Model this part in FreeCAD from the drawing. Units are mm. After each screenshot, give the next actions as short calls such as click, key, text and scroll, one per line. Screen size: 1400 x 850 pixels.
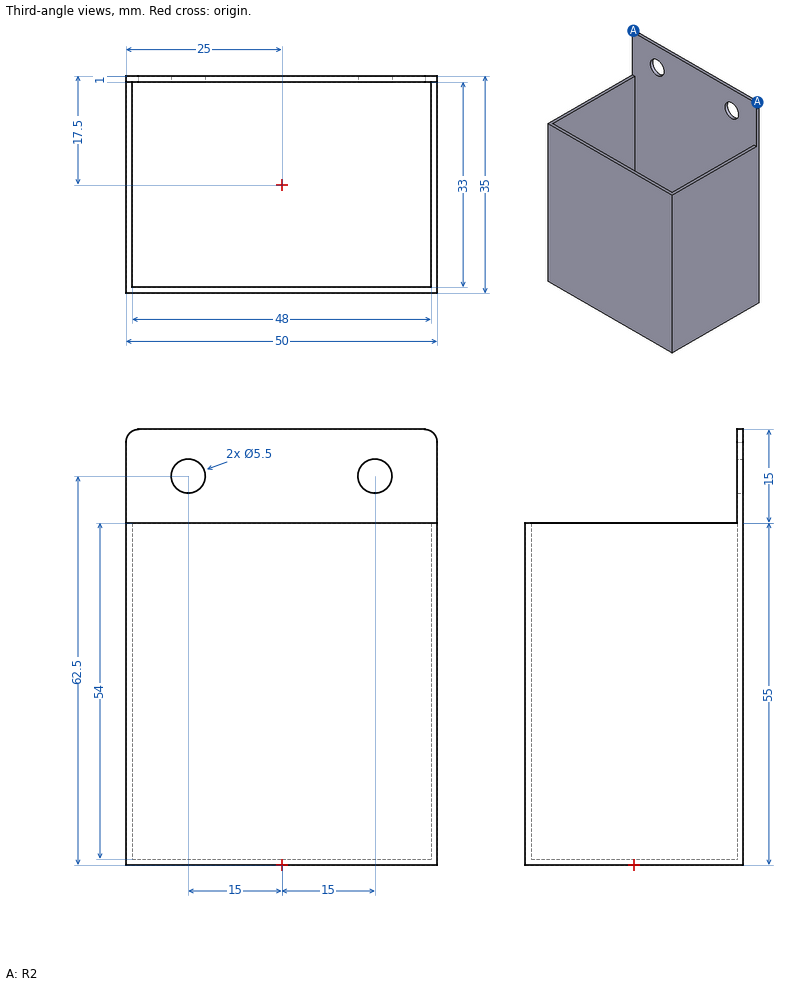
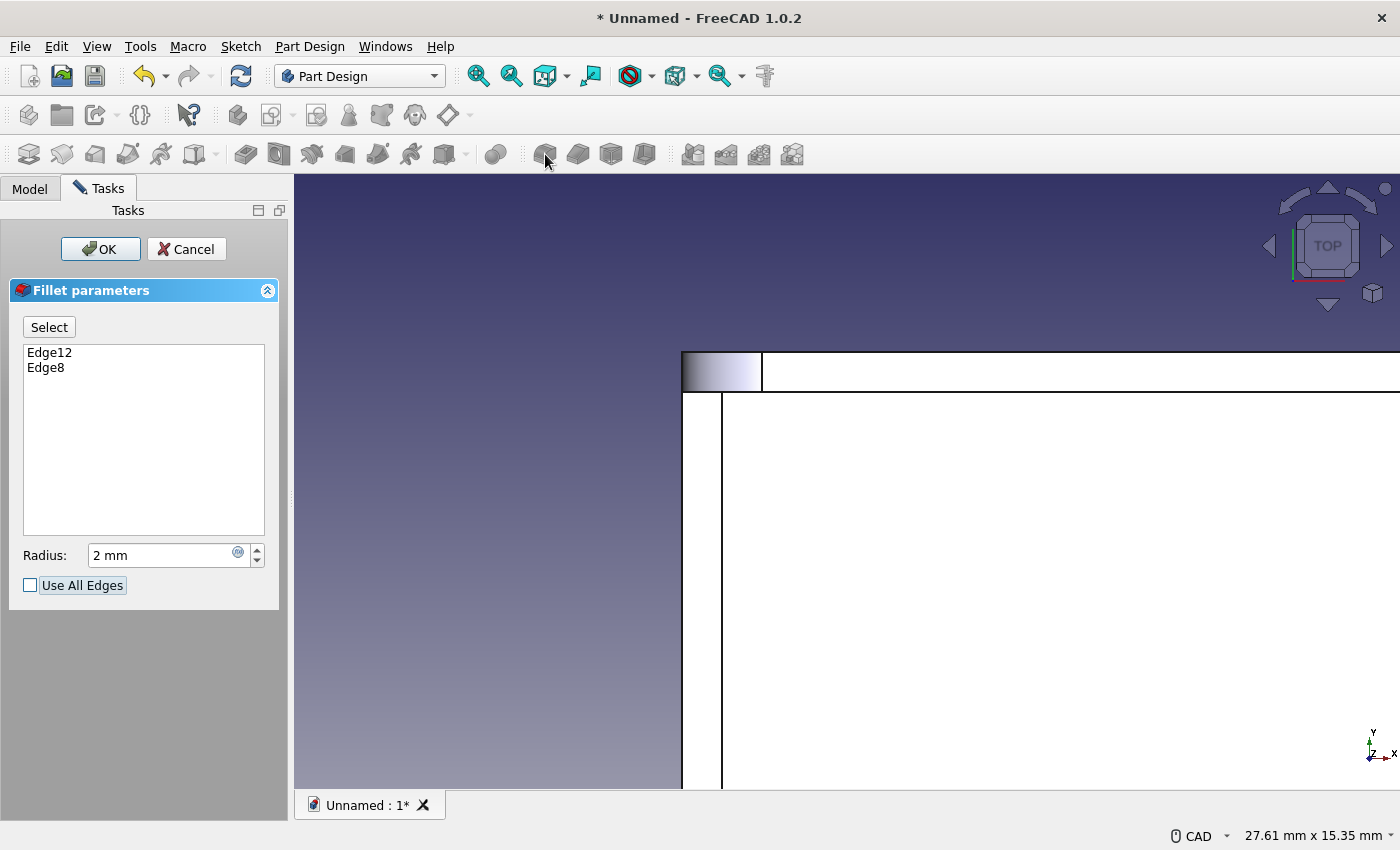
click(101, 249)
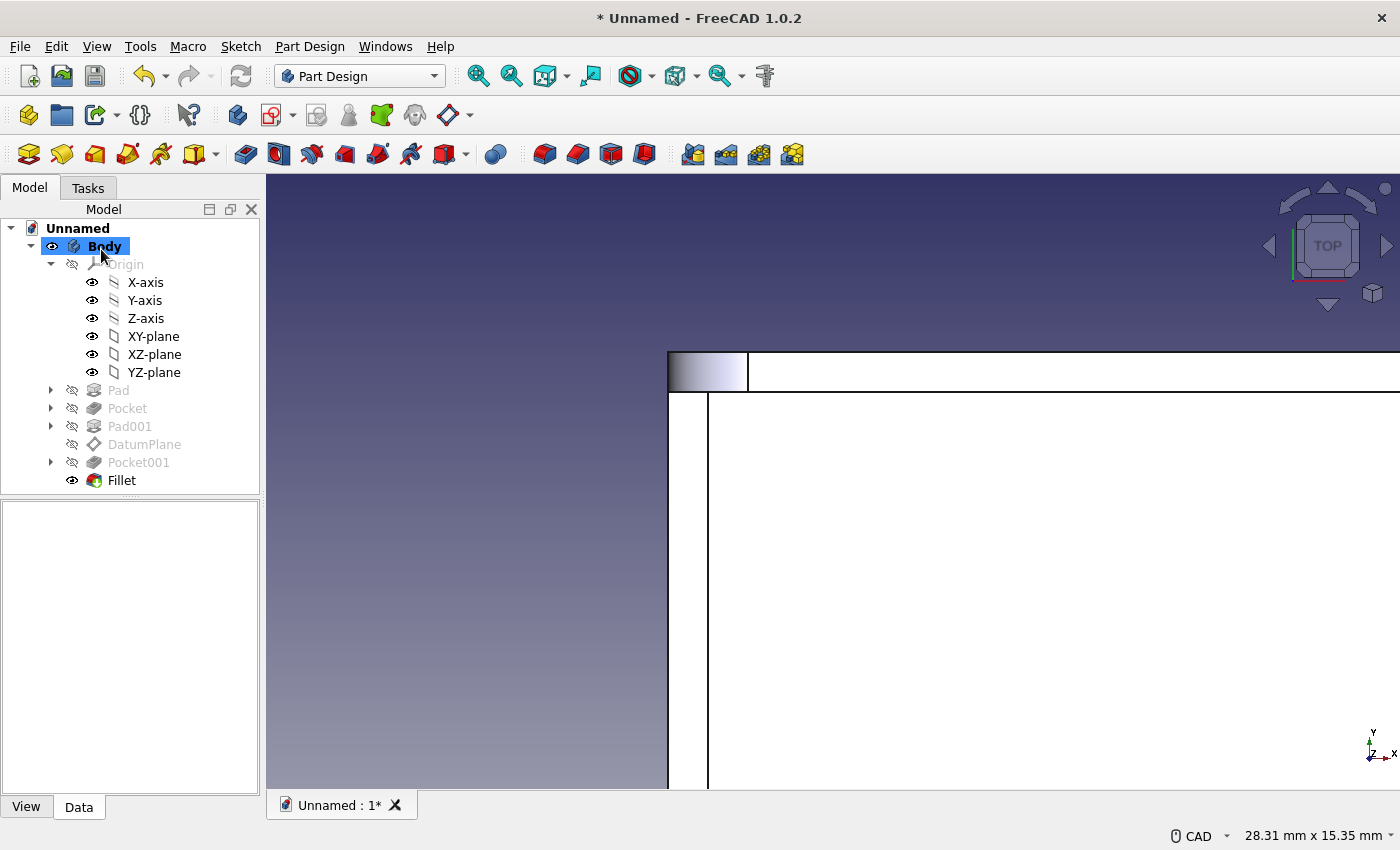
key(0)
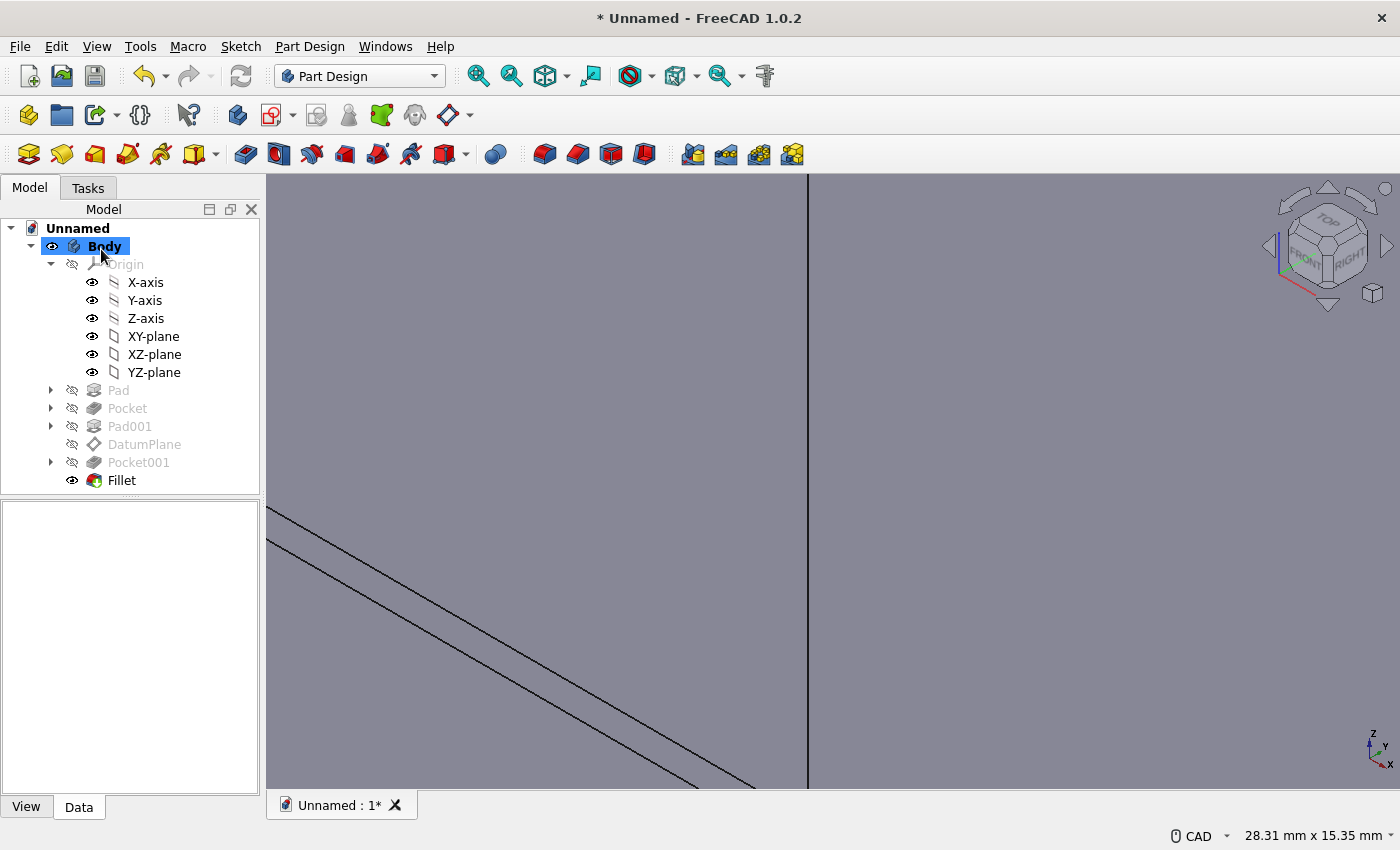
key(v)
key(f)